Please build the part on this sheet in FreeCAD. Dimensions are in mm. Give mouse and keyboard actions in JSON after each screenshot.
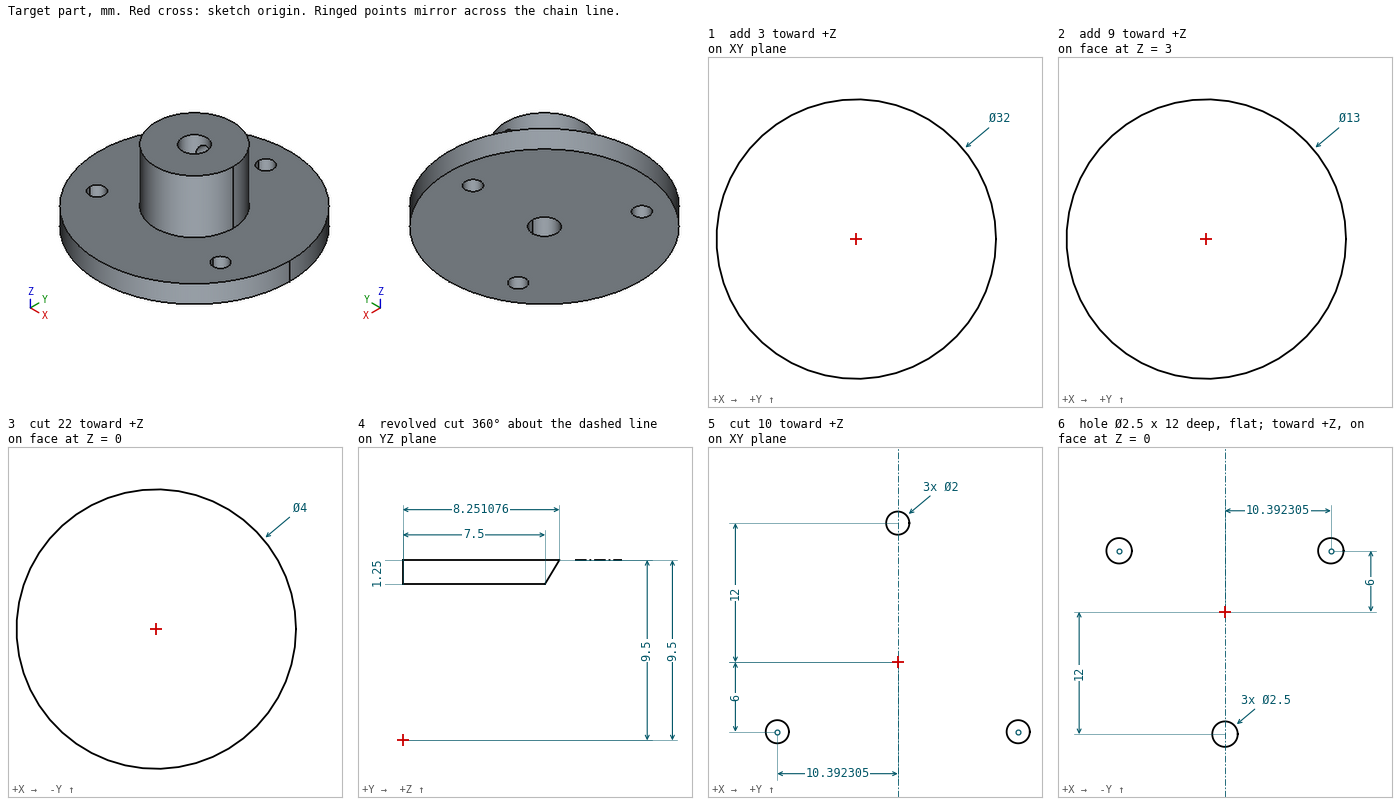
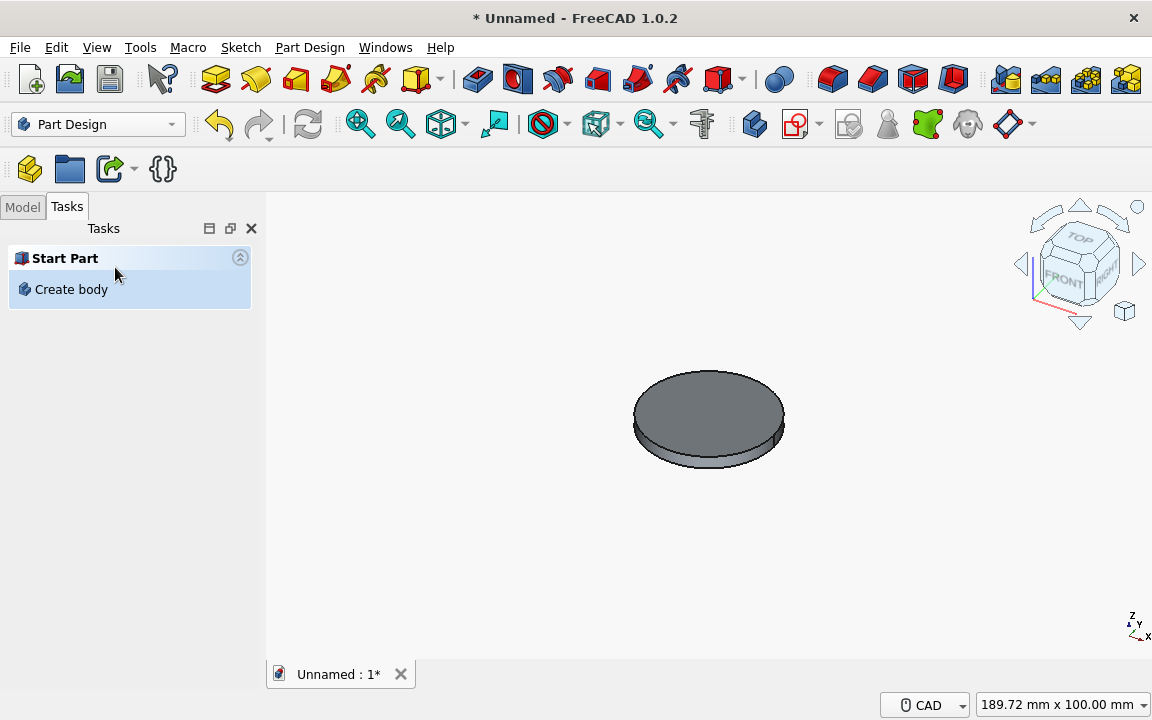
{"action": "left_click", "coordinate": [362, 124]}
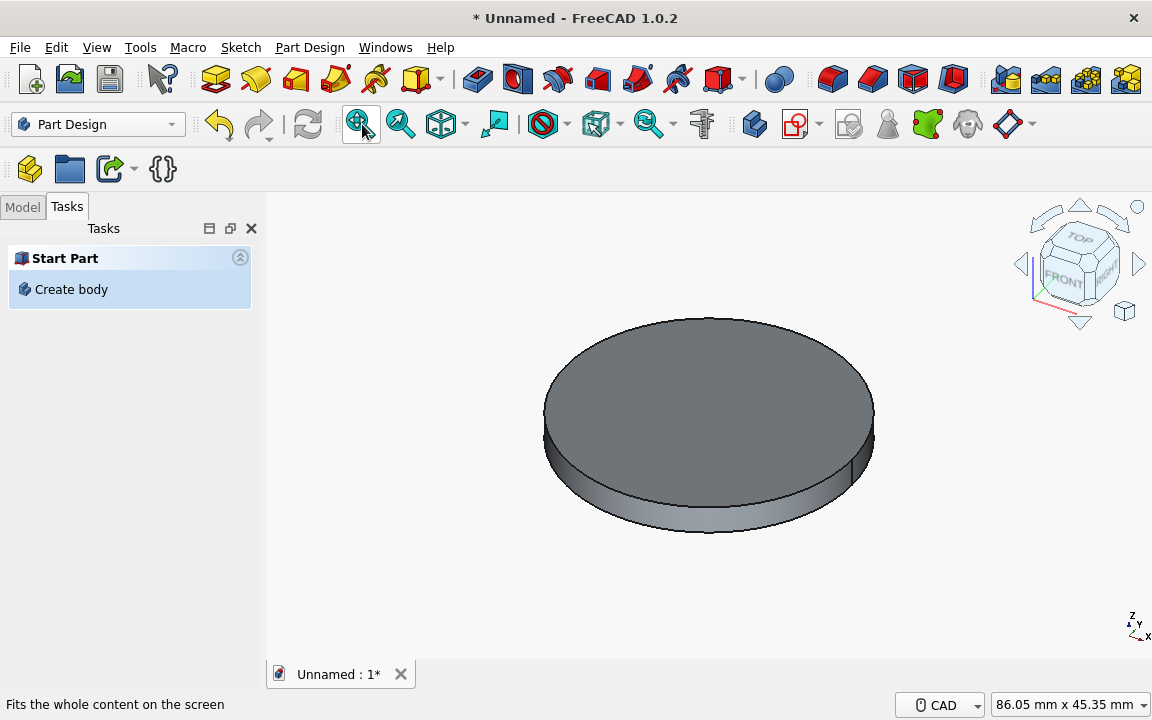
{"action": "left_click", "coordinate": [709, 412]}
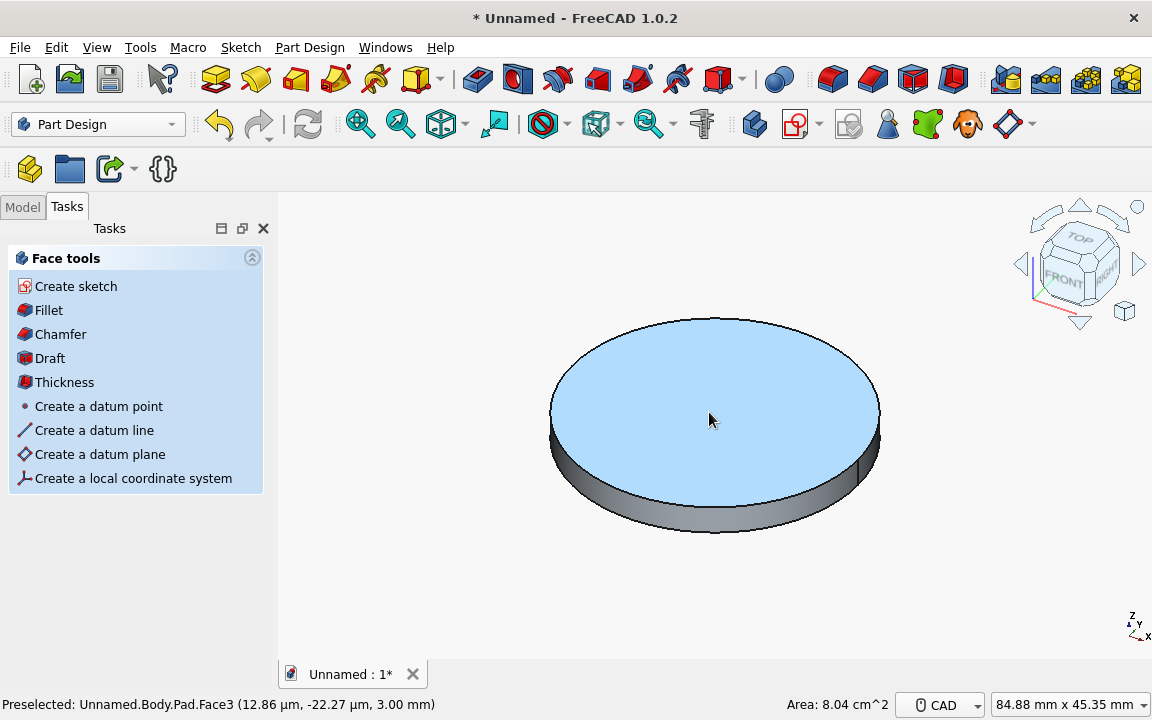
{"action": "left_click", "coordinate": [796, 124]}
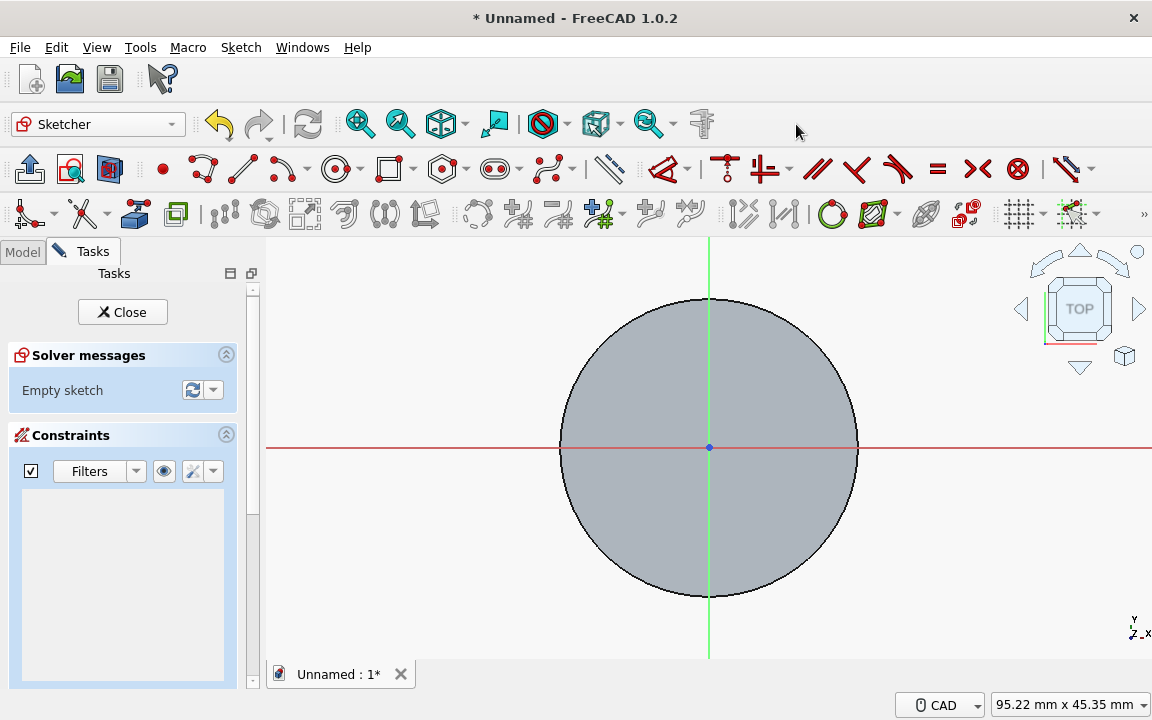
{"action": "scroll", "coordinate": [765, 448], "scroll_direction": "up", "scroll_amount": 4}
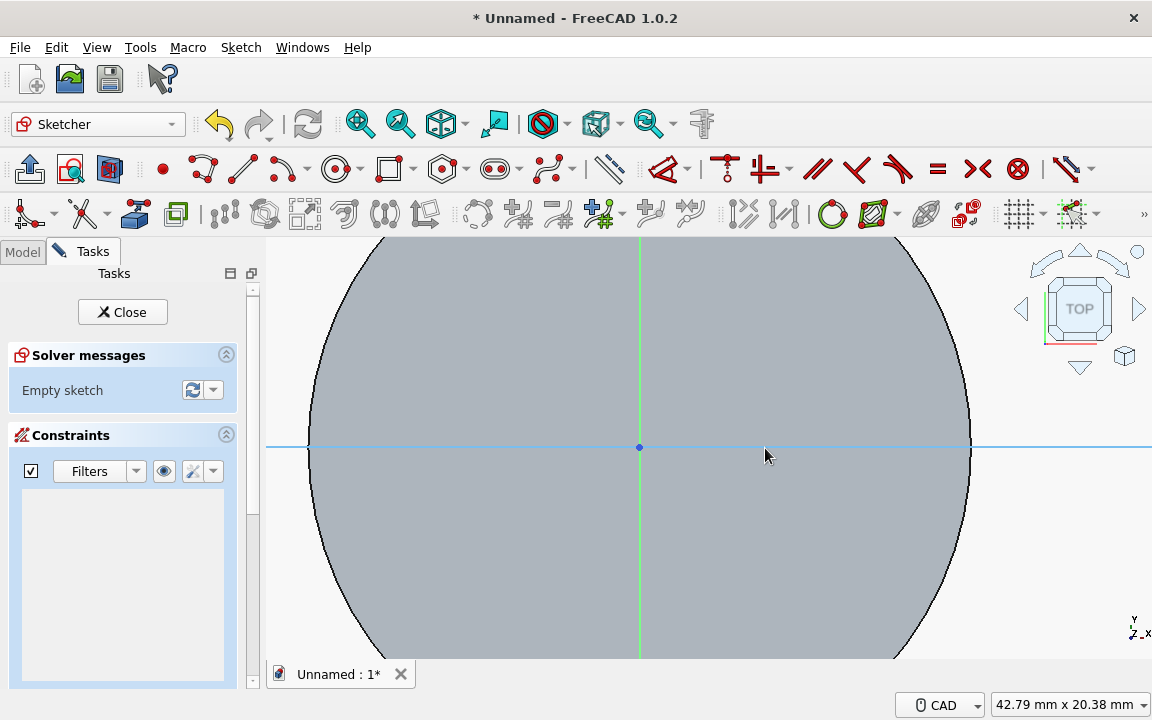
{"action": "left_click", "coordinate": [336, 170]}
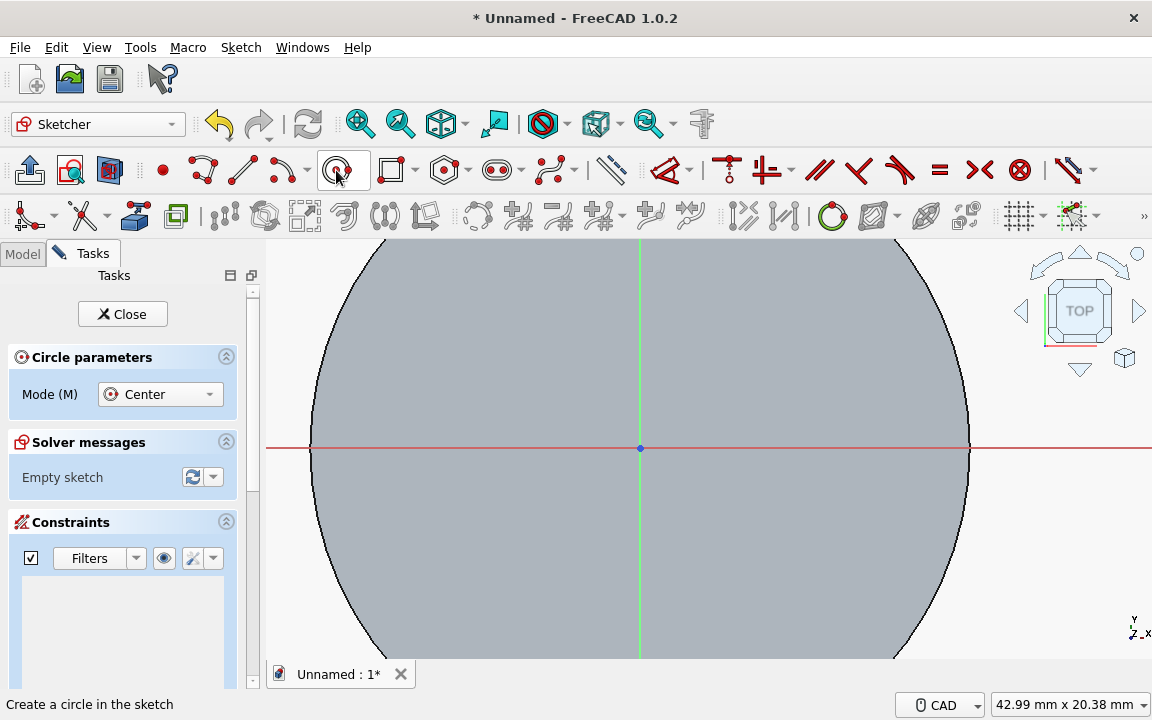
{"action": "left_click", "coordinate": [640, 448]}
{"action": "mouse_move", "coordinate": [735, 354]}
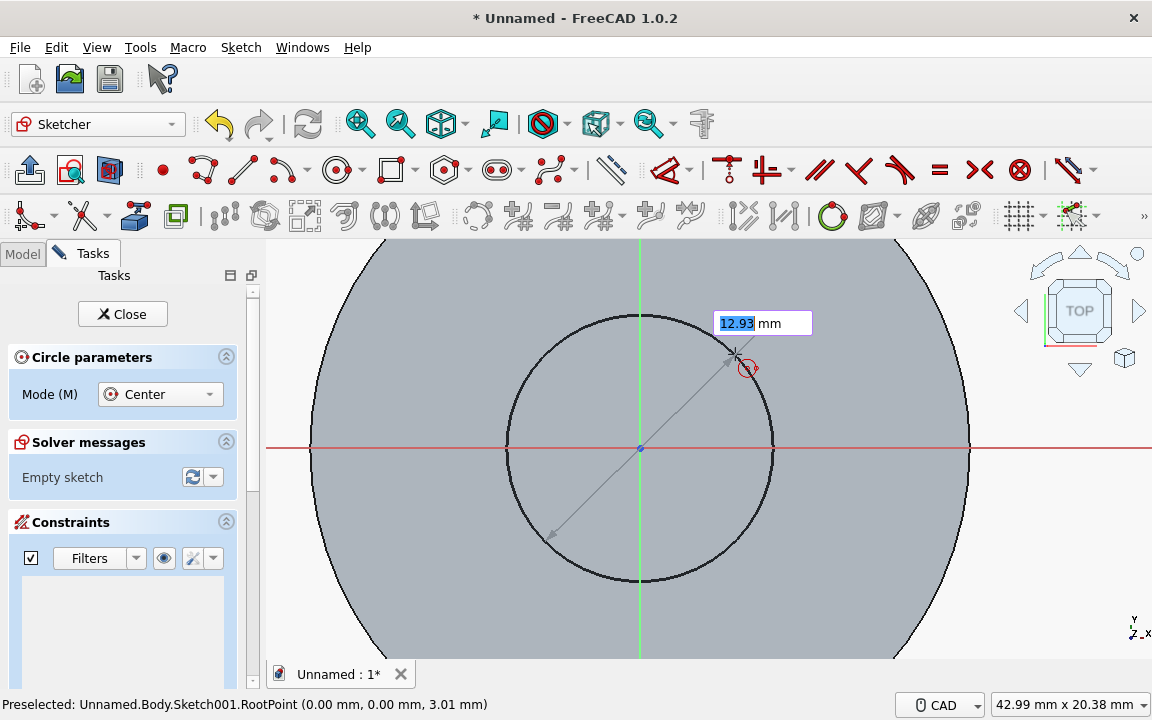
{"action": "type", "text": "13"}
{"action": "key", "text": "Return"}
{"action": "key", "text": "Escape"}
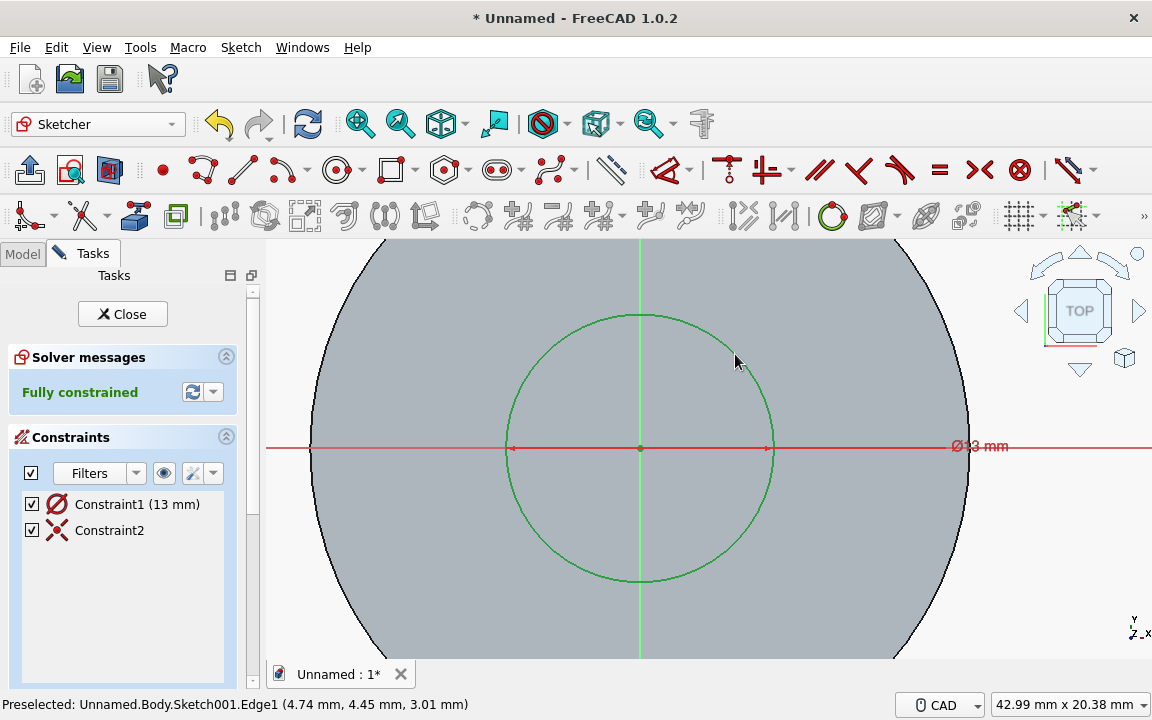
{"action": "left_click", "coordinate": [123, 314]}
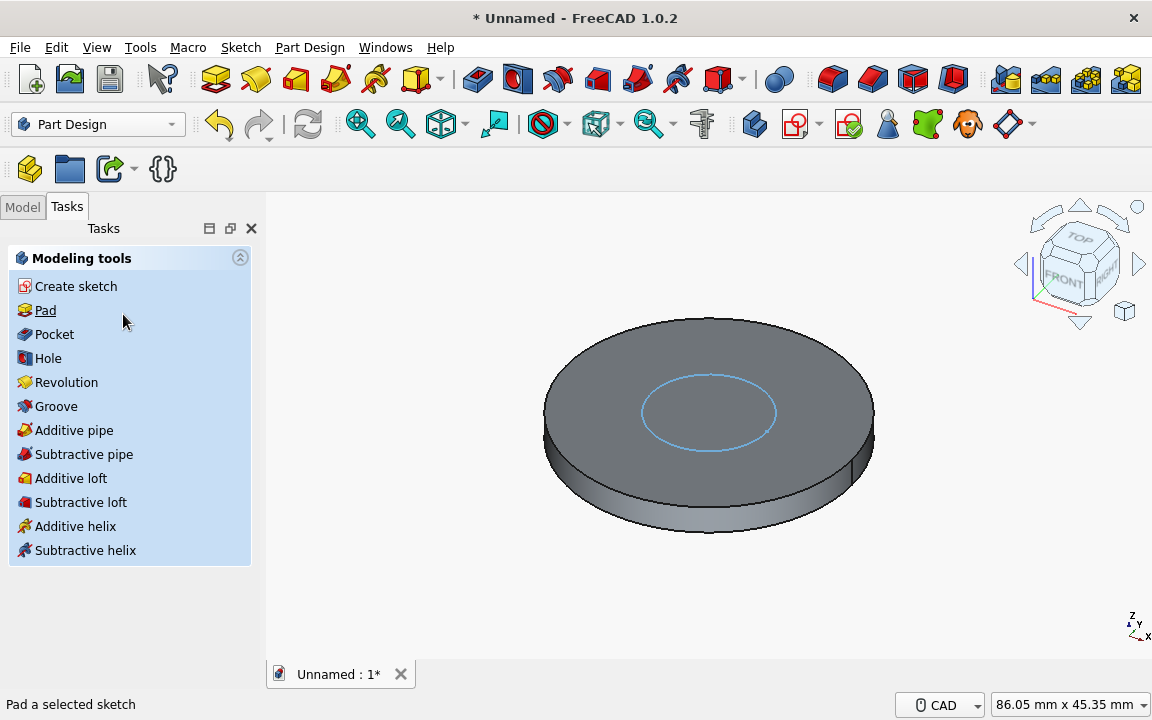
{"action": "left_click", "coordinate": [216, 80]}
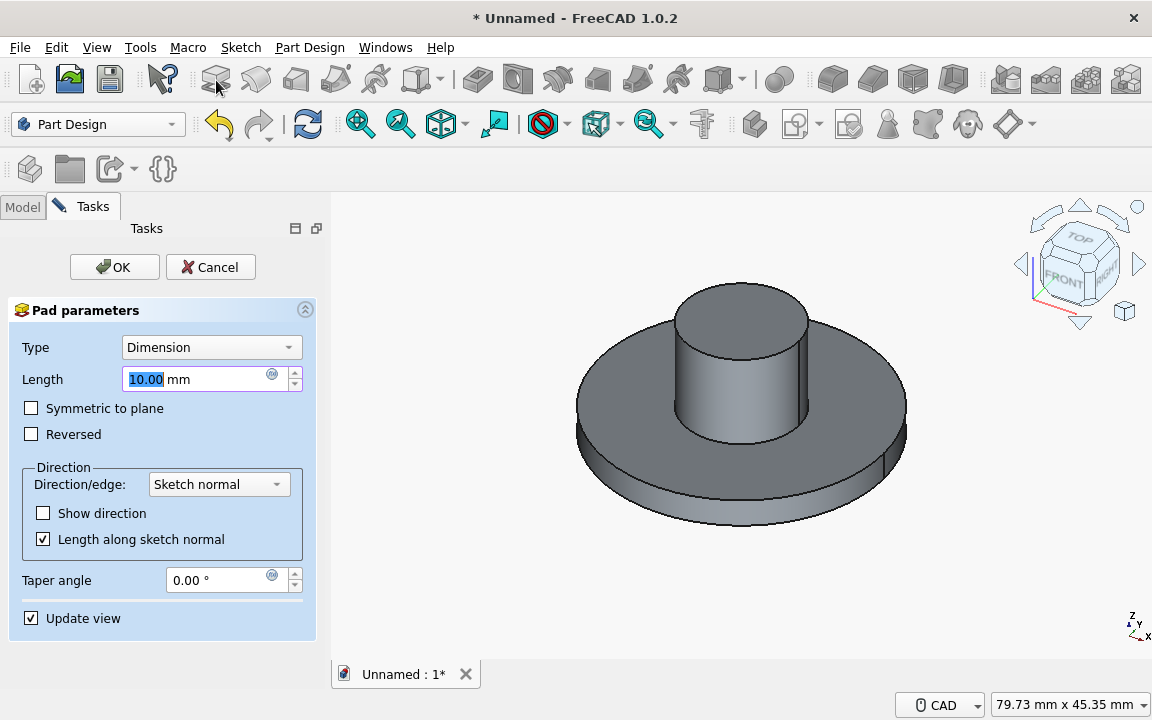
{"action": "type", "text": "9"}
{"action": "key", "text": "Tab"}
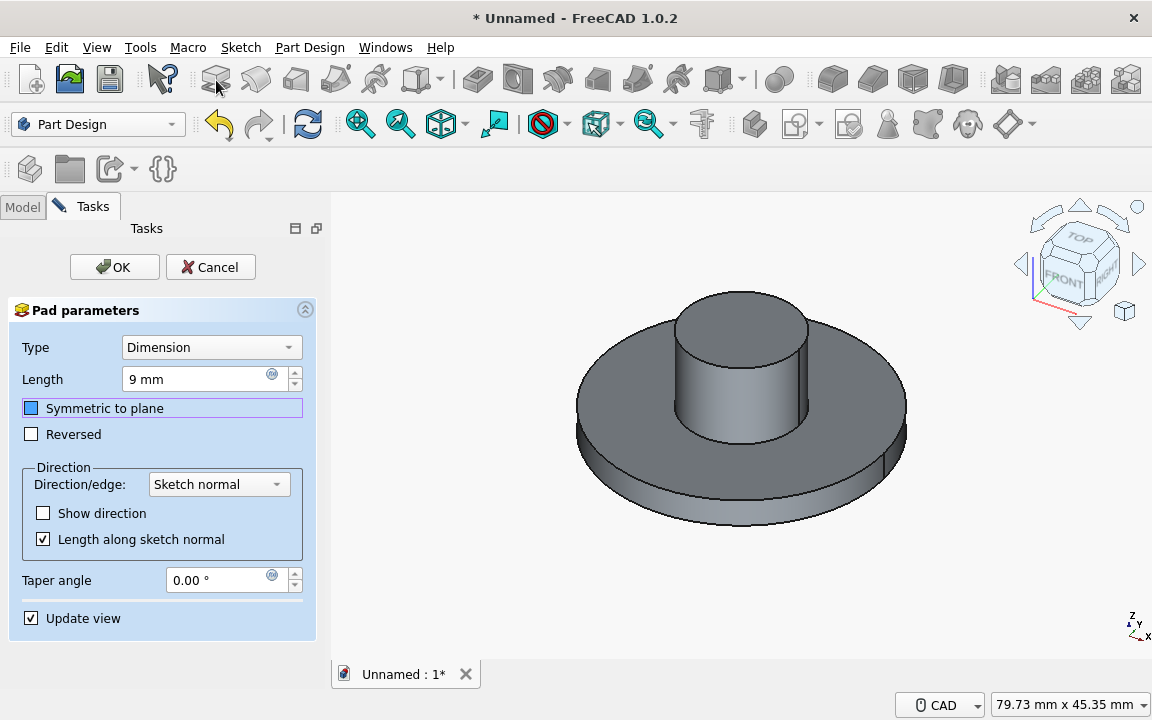
{"action": "left_click", "coordinate": [115, 267]}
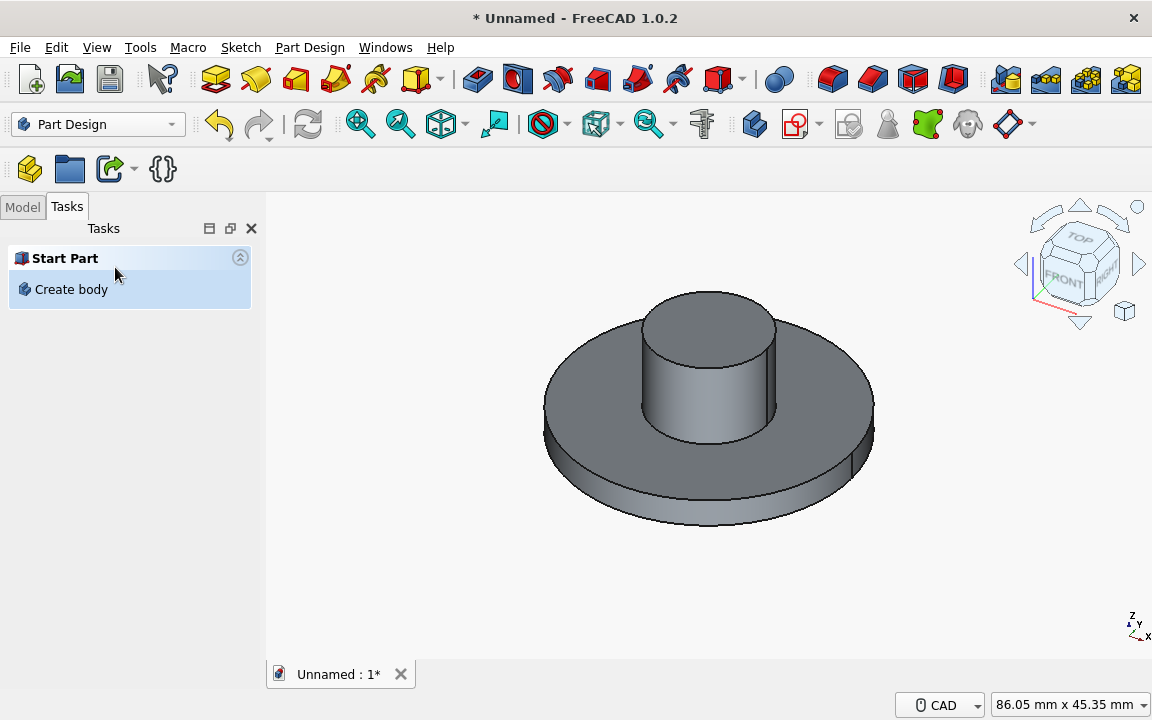
{"action": "key", "text": "5"}